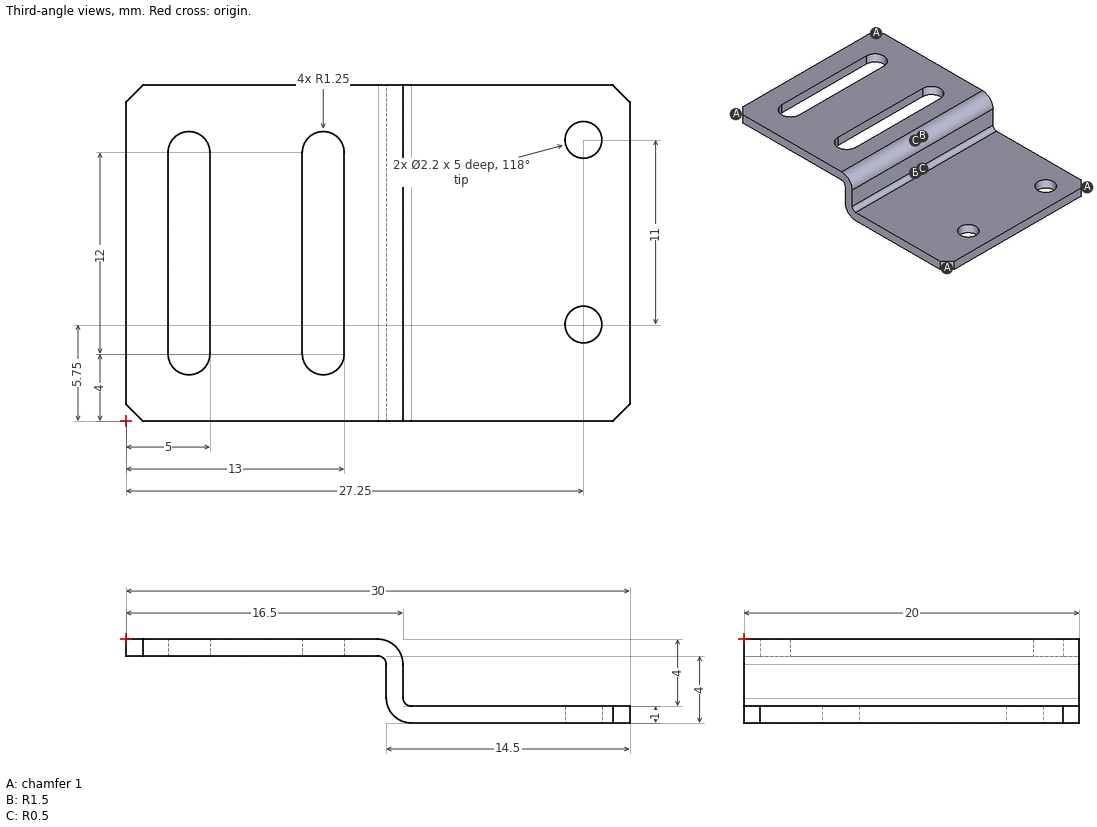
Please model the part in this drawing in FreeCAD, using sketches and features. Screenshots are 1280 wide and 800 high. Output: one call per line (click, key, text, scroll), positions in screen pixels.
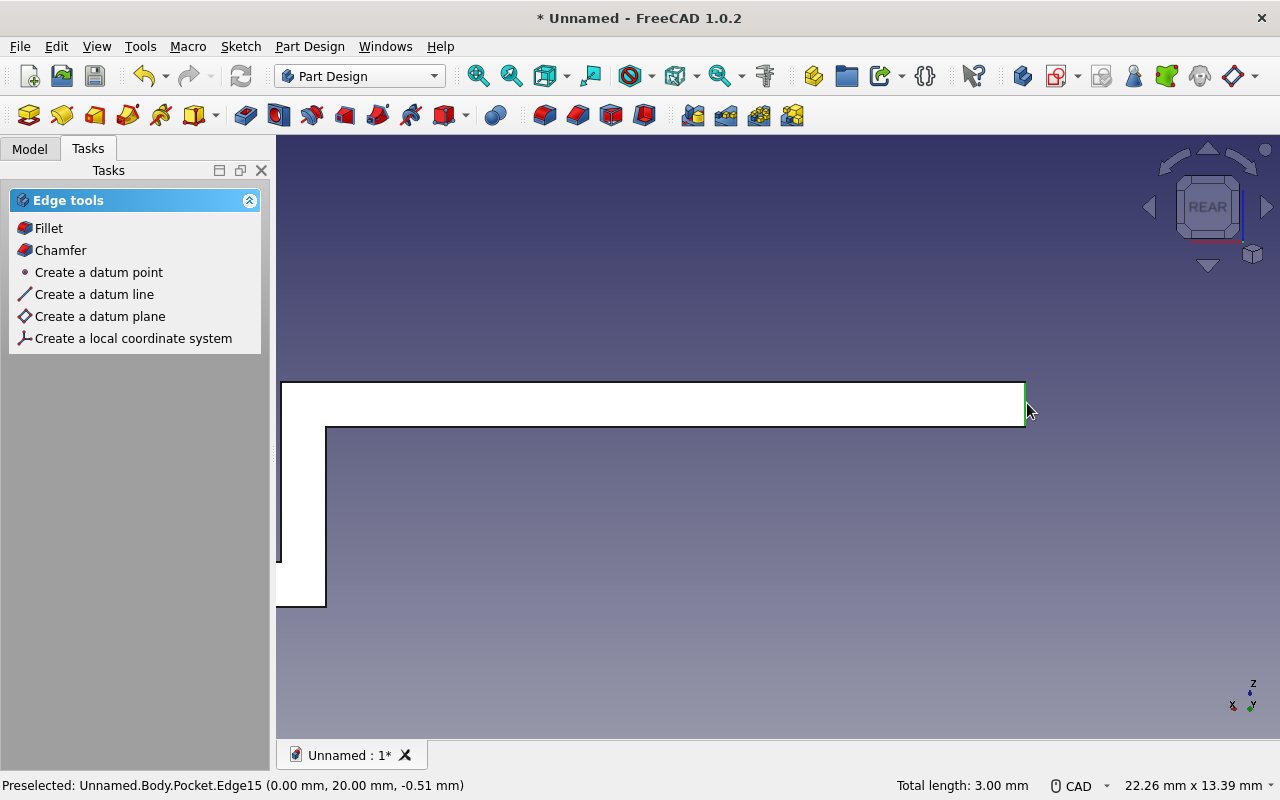
click(479, 76)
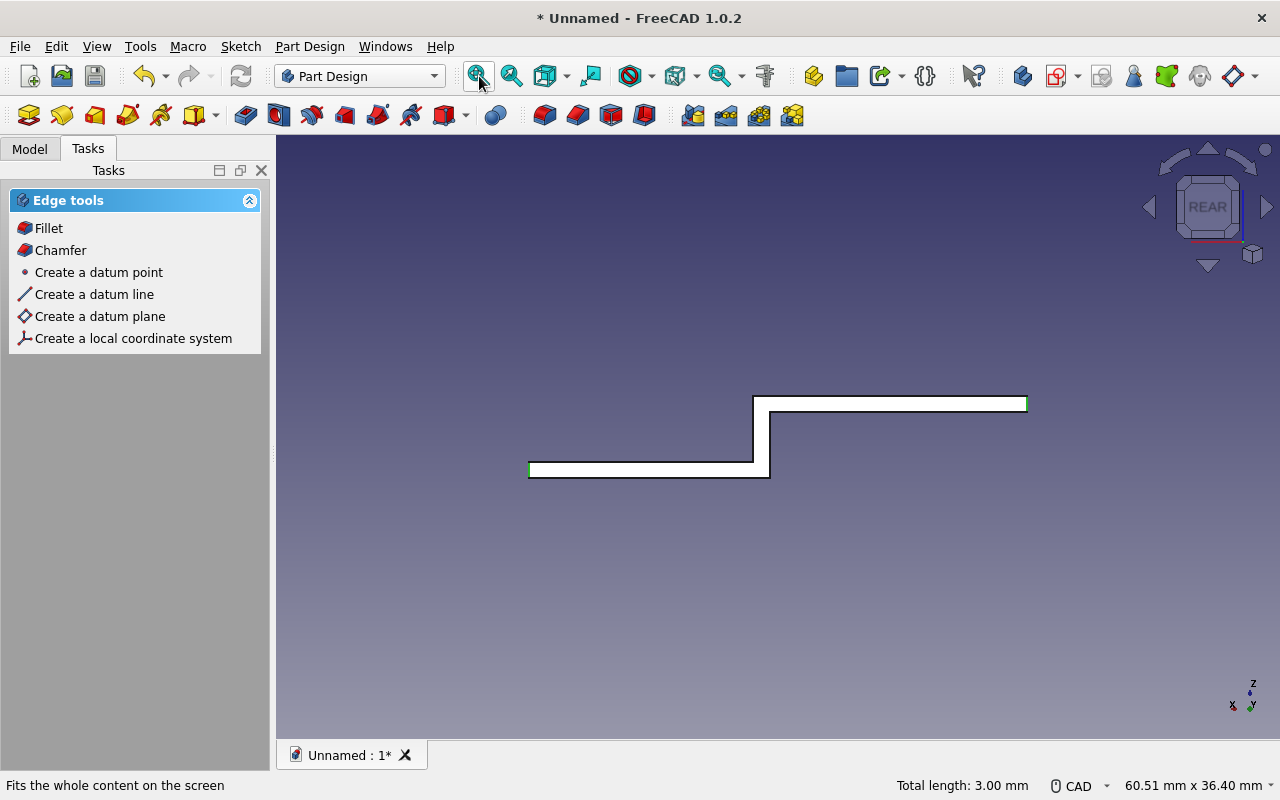
key(6)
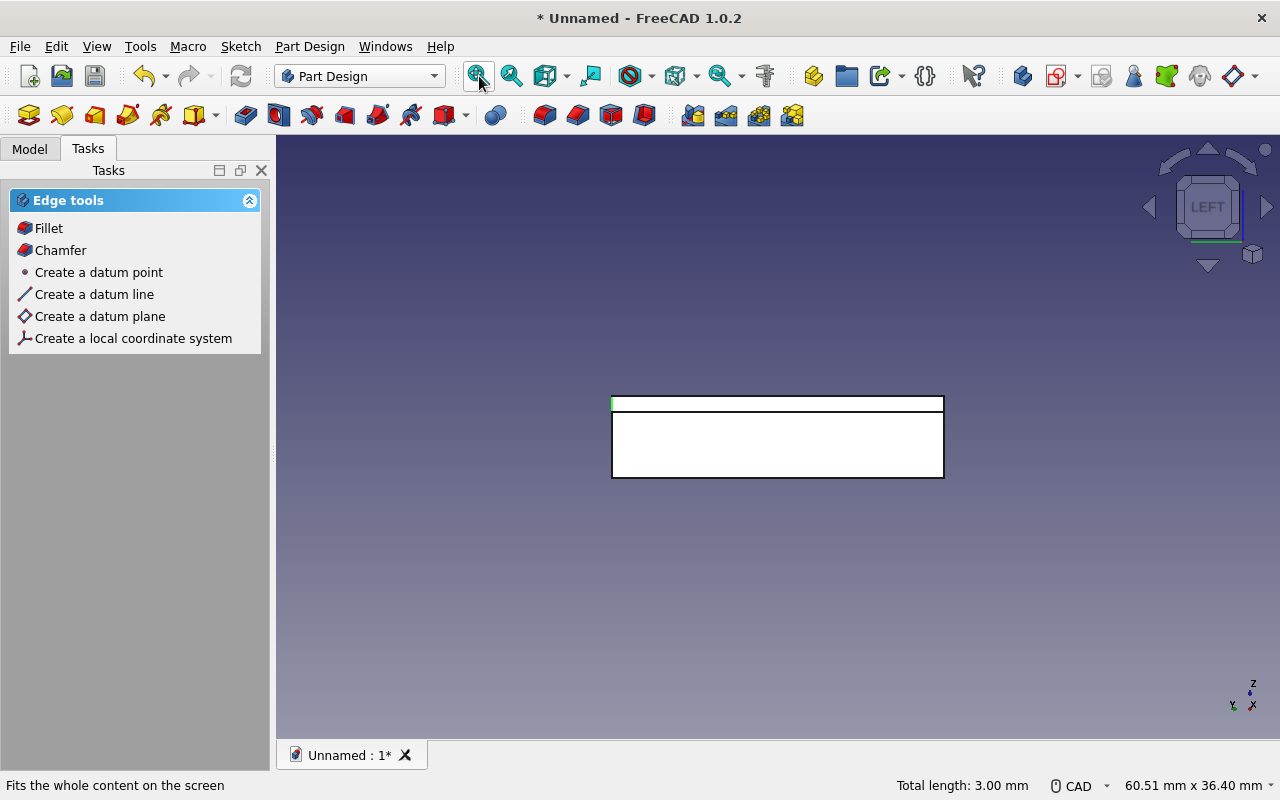
click(479, 76)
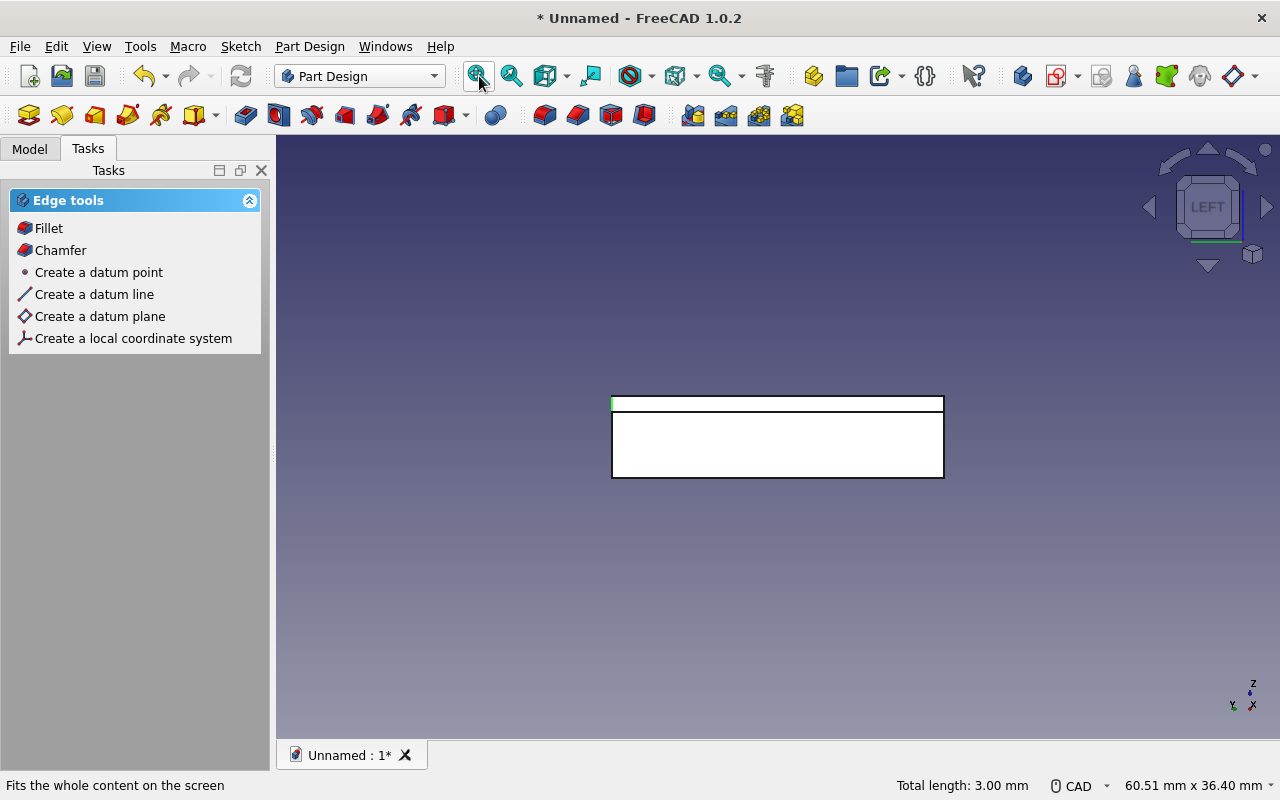
click(944, 403, ctrl)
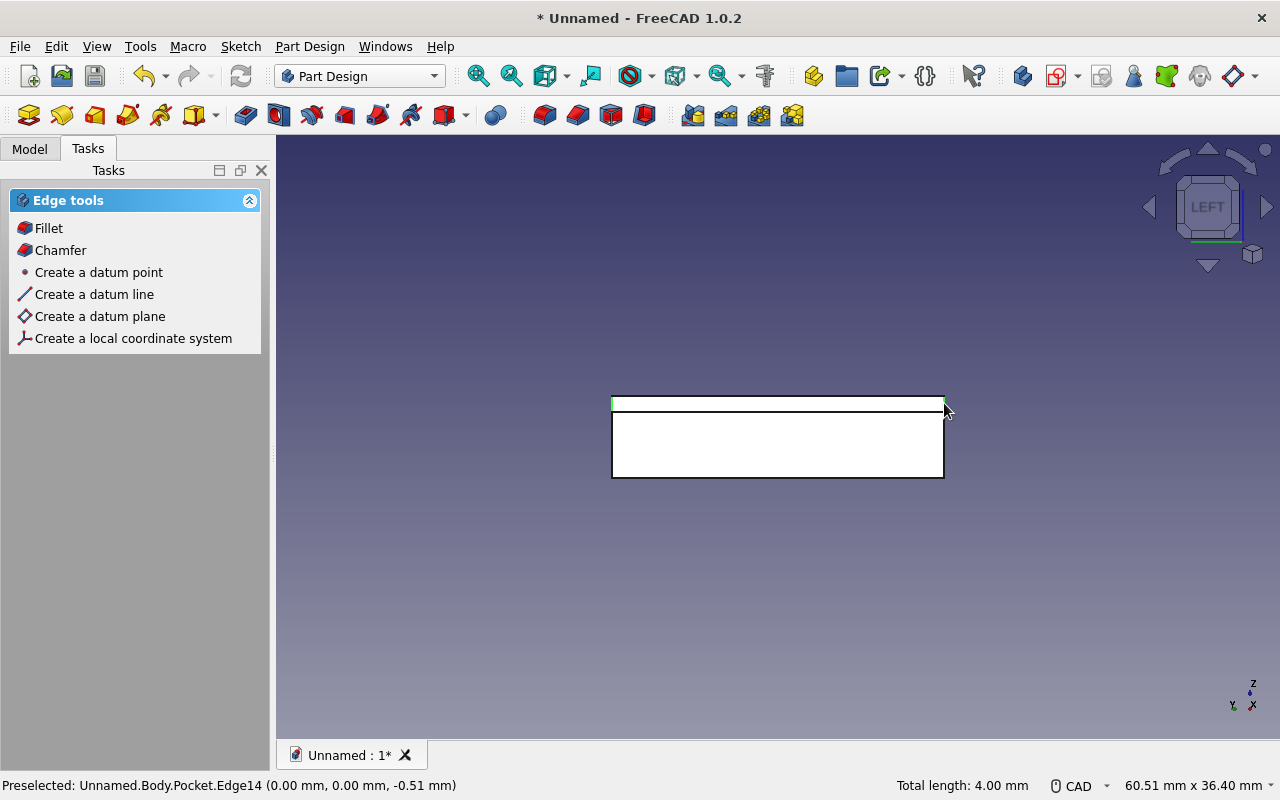
click(578, 116)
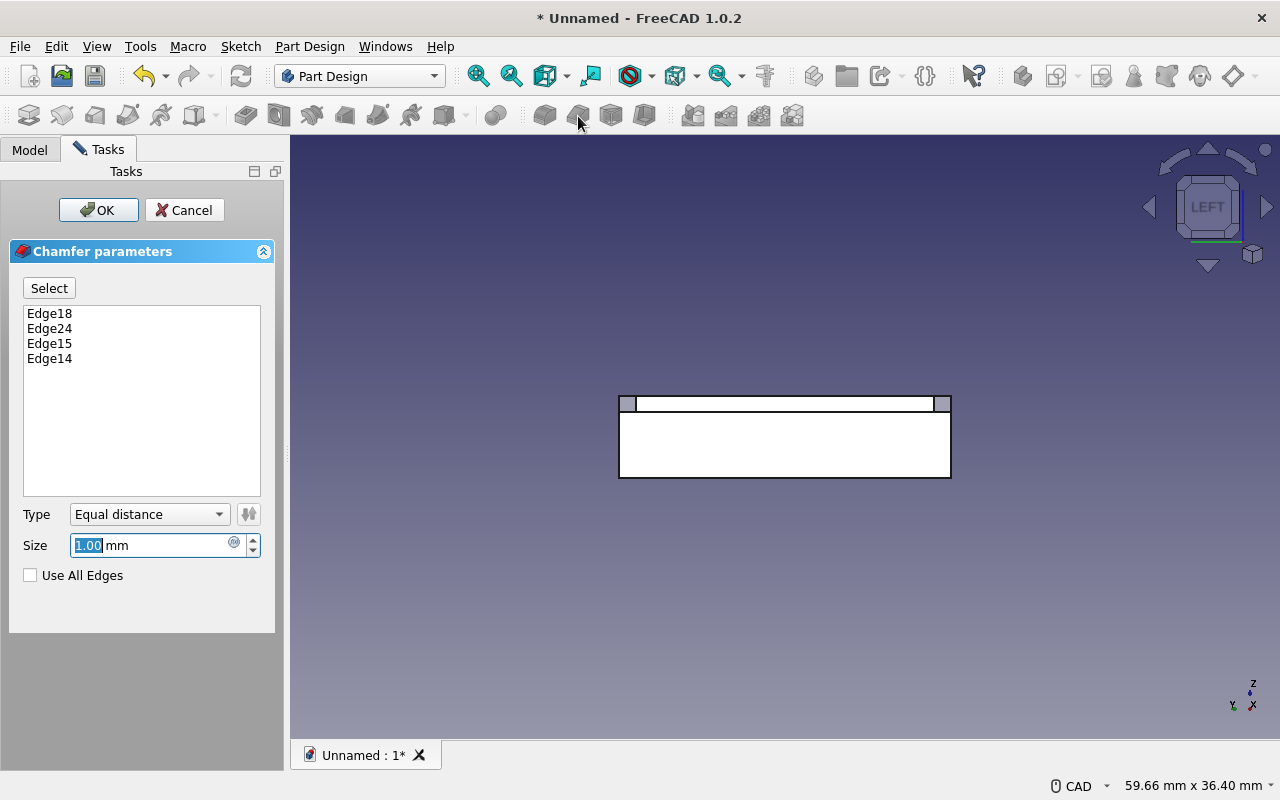
text(1)
key(Tab)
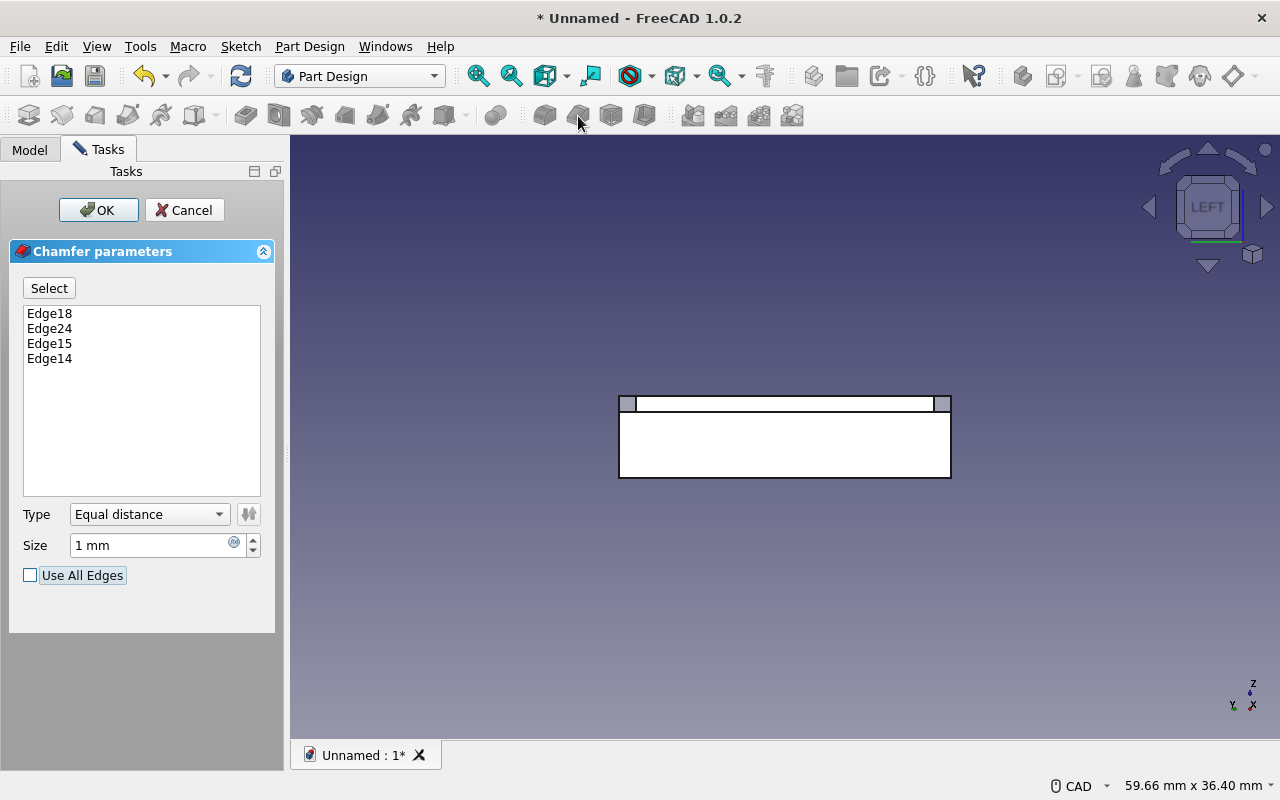
click(99, 210)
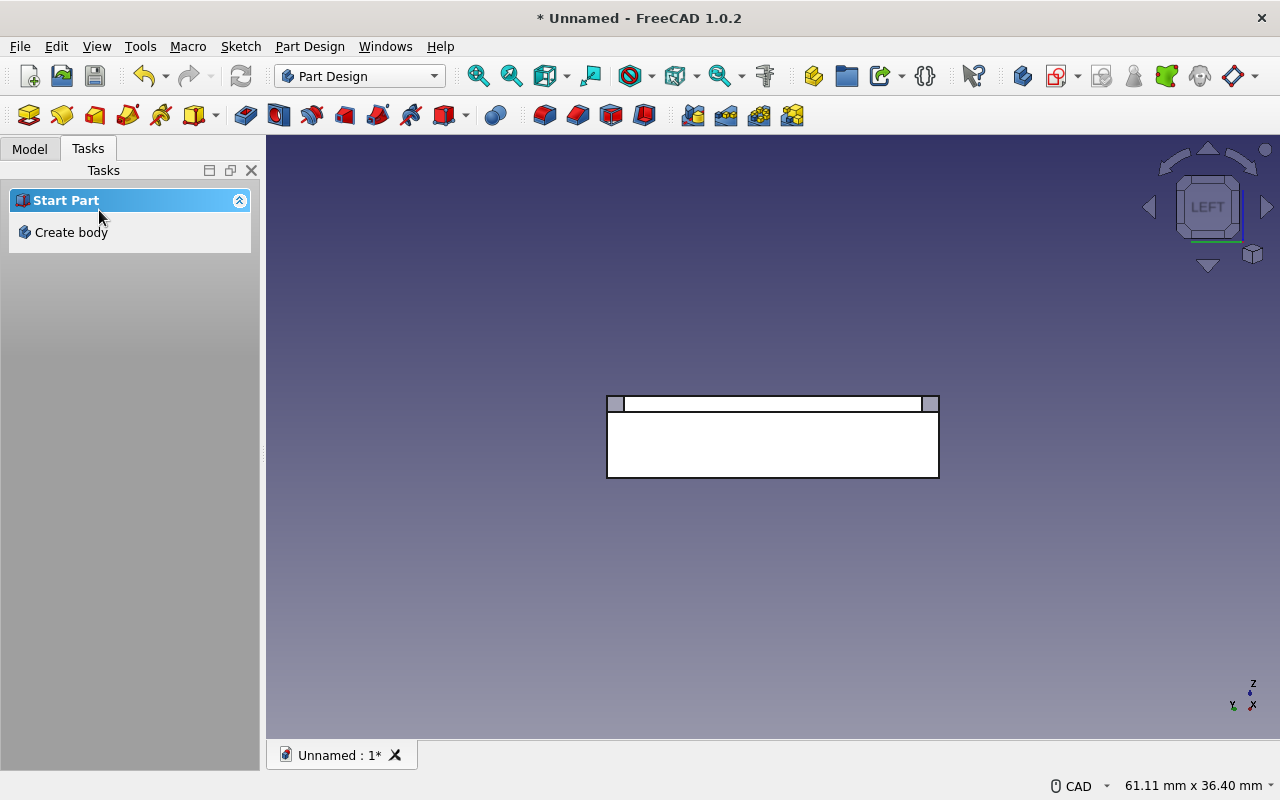
click(479, 76)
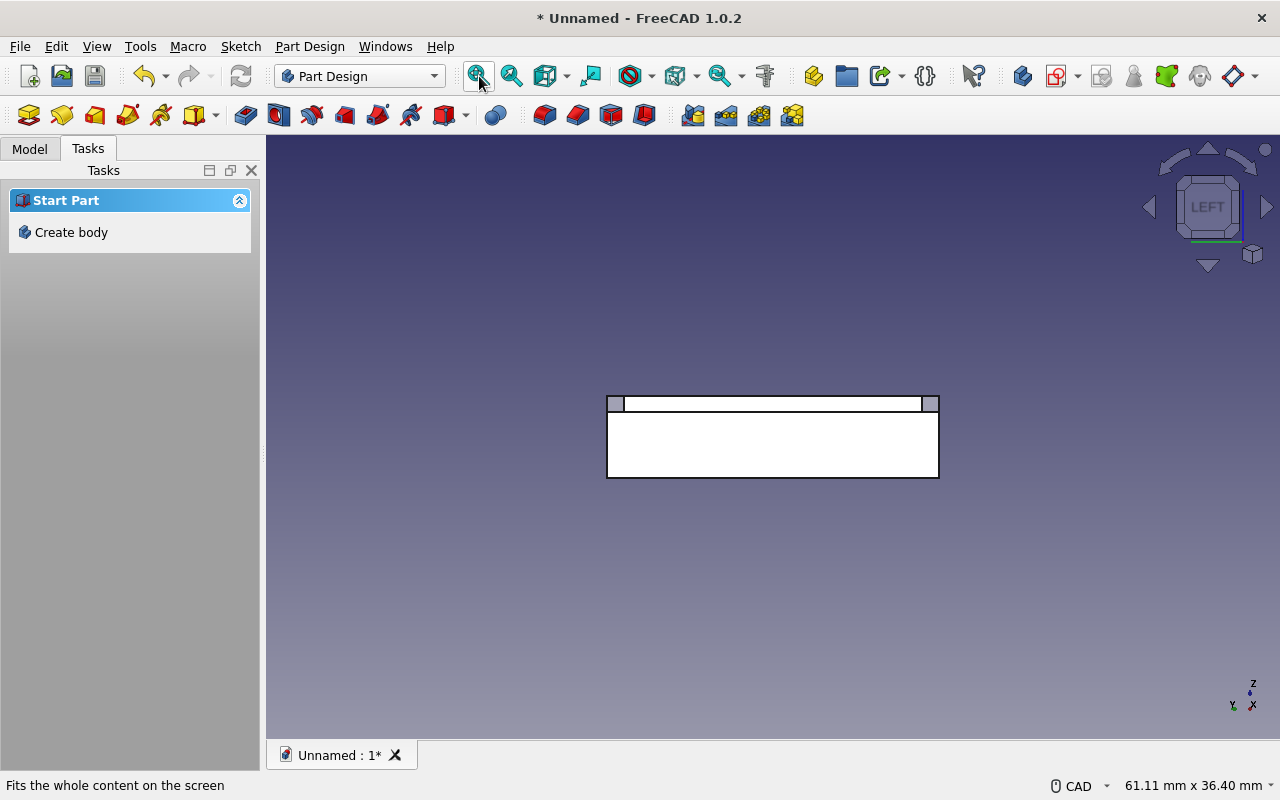
click(773, 477)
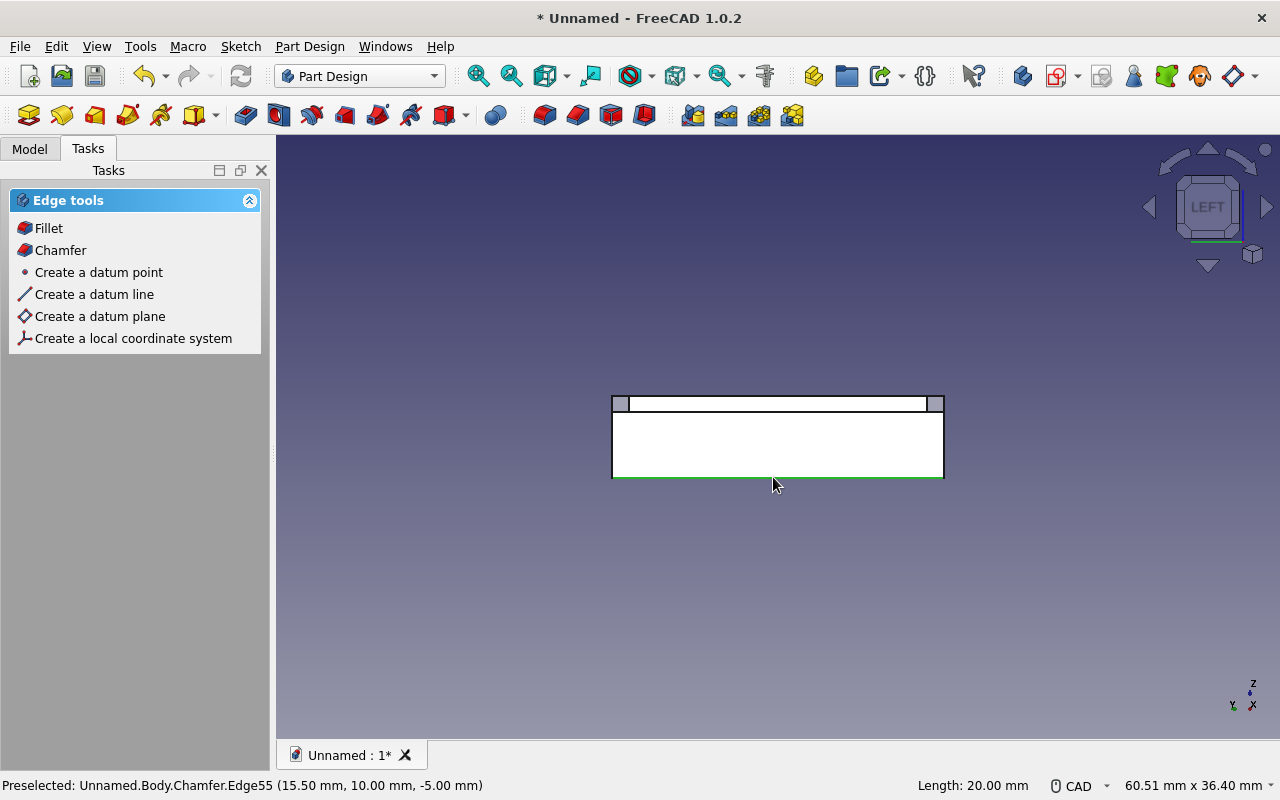
key(0)